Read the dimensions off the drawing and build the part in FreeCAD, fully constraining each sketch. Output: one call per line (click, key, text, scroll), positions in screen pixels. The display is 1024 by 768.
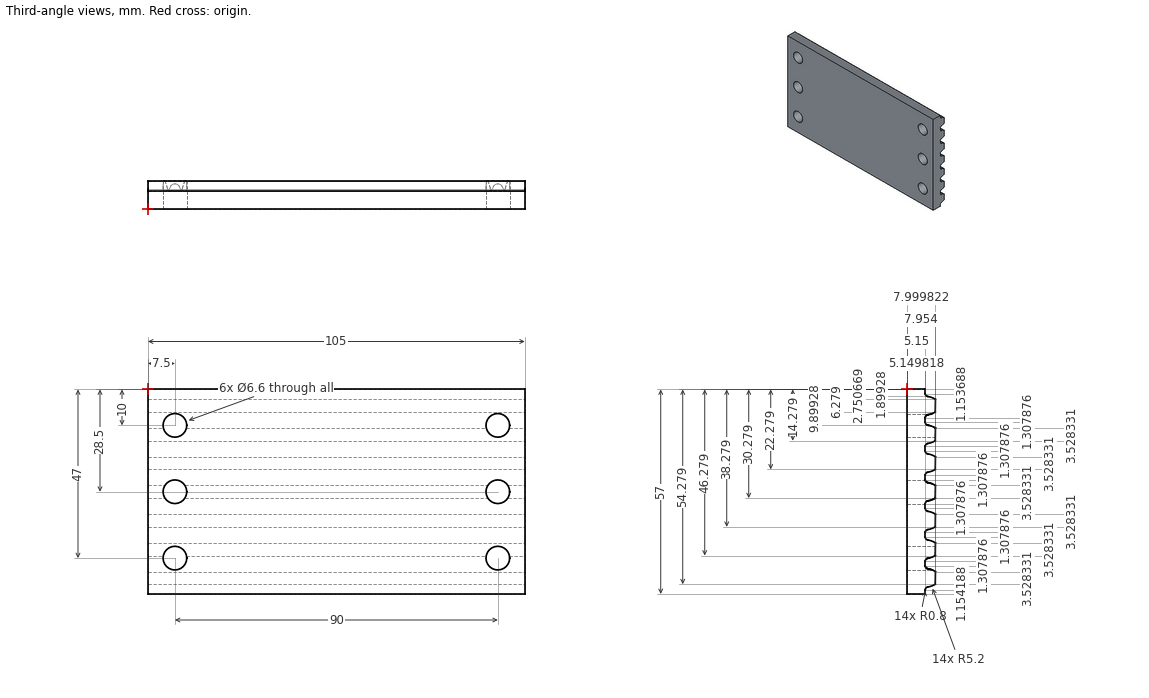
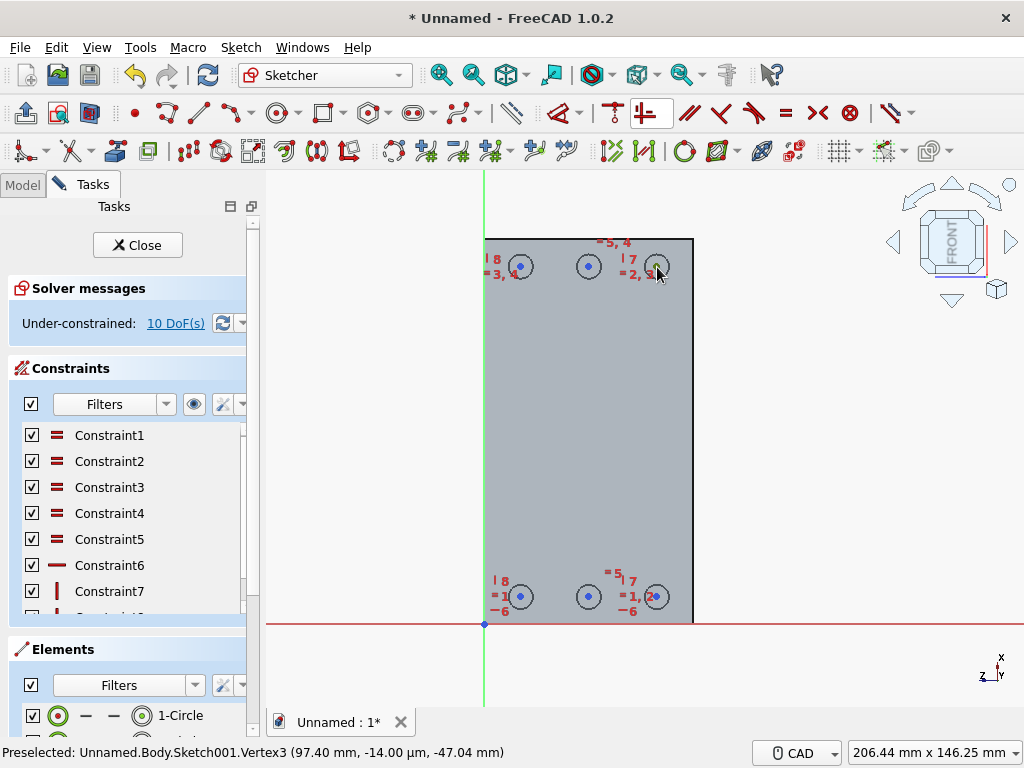
click(521, 267)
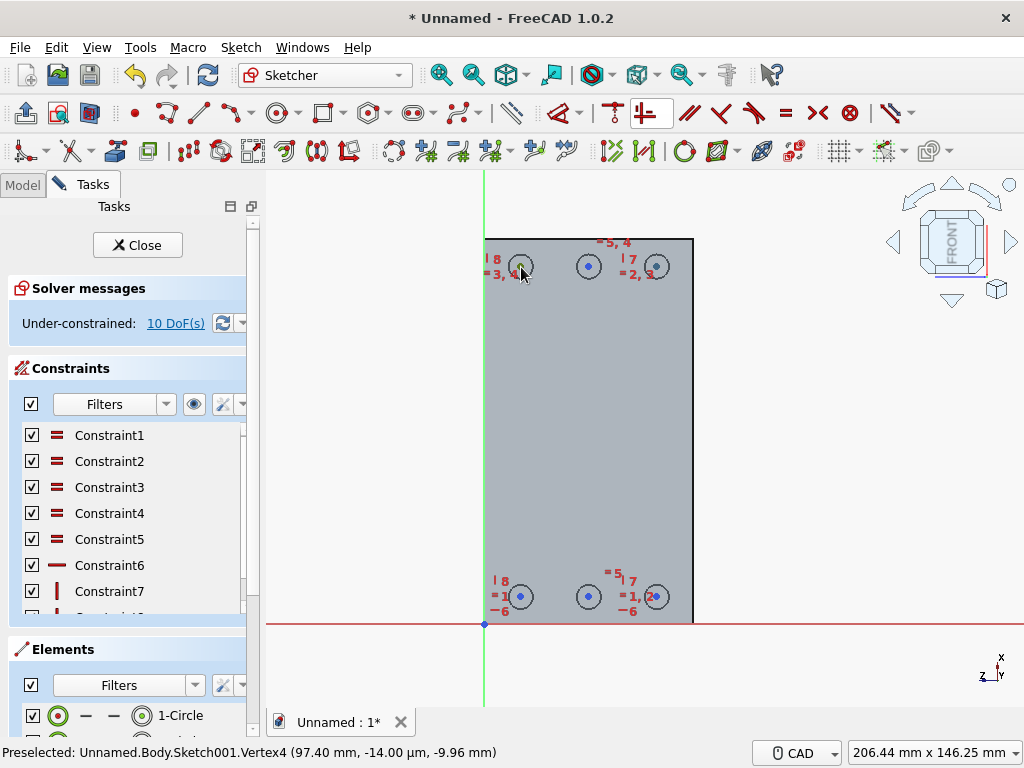
click(668, 114)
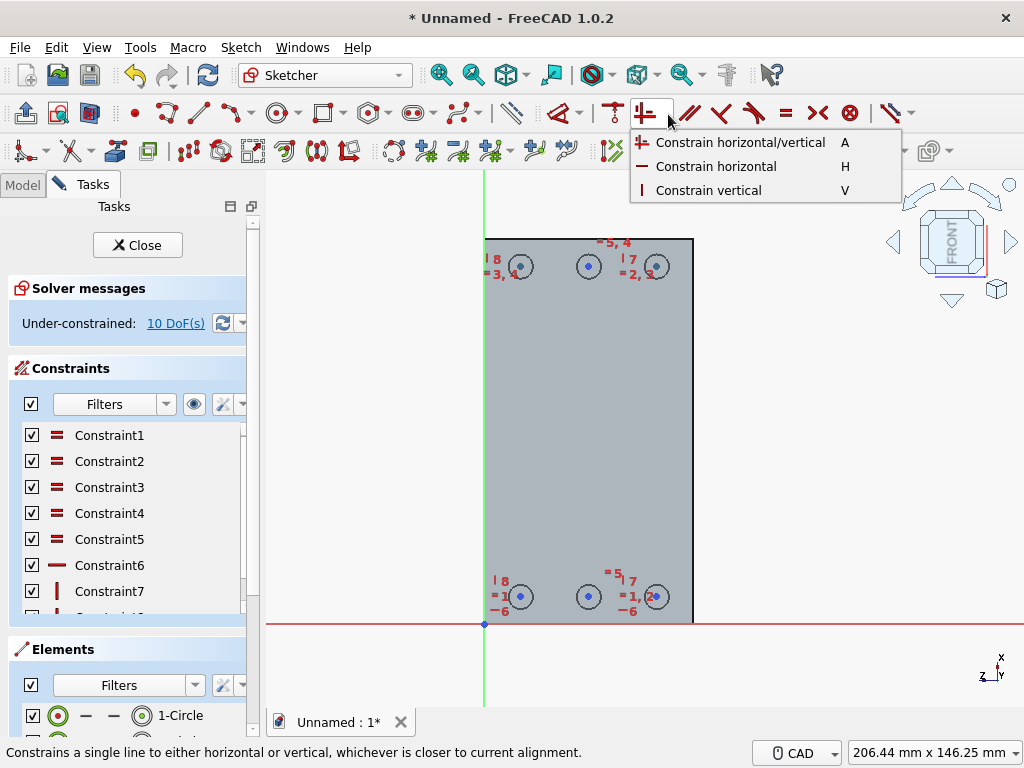
click(766, 166)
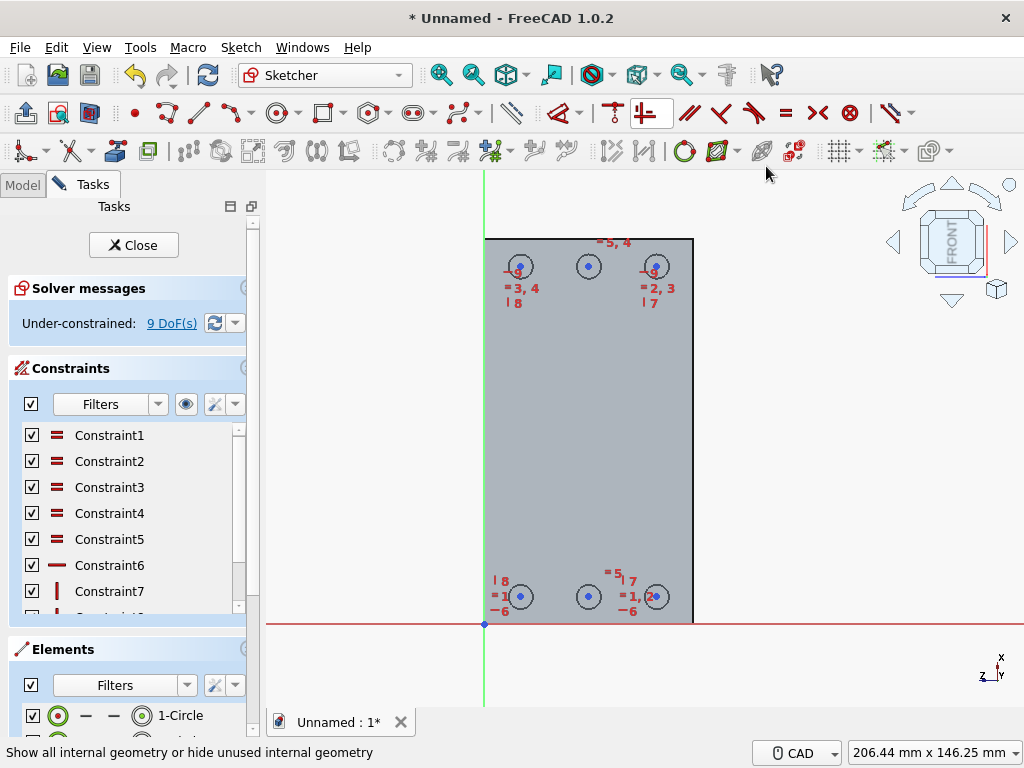
click(657, 267)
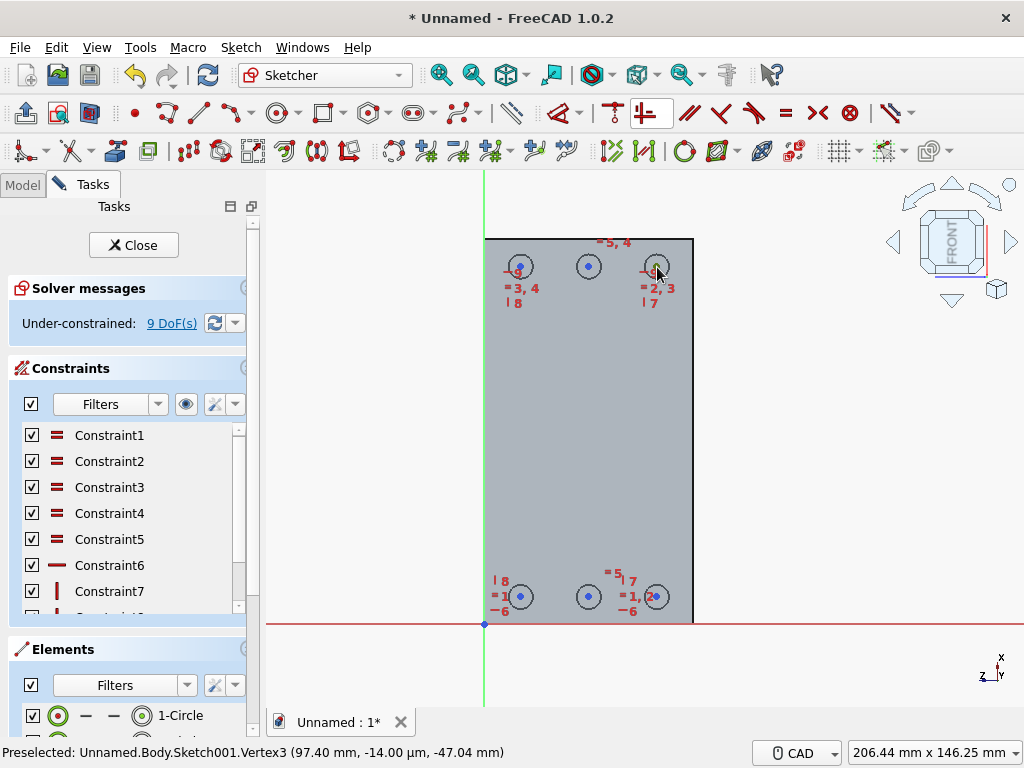
click(589, 267)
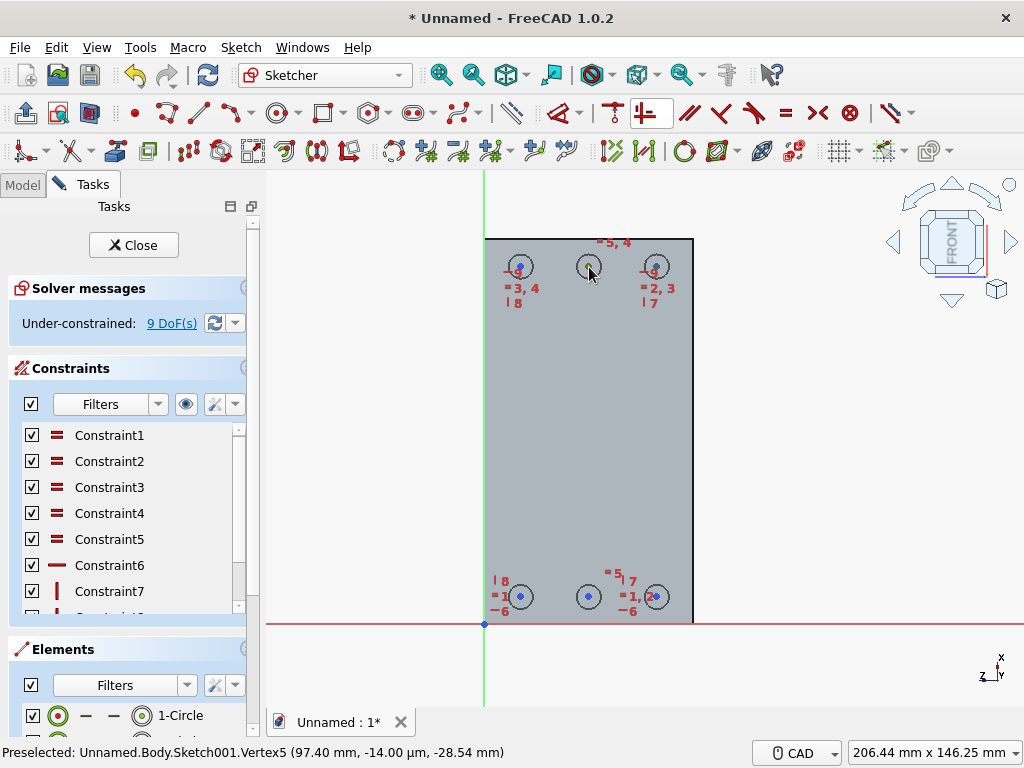
key(h)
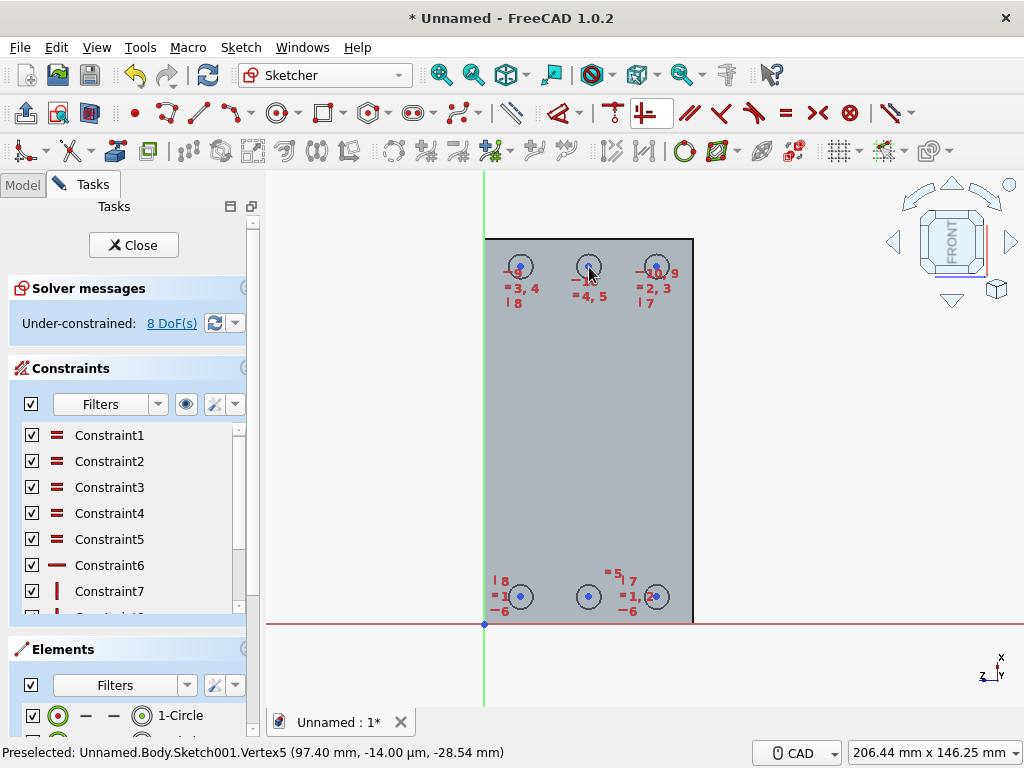
click(589, 267)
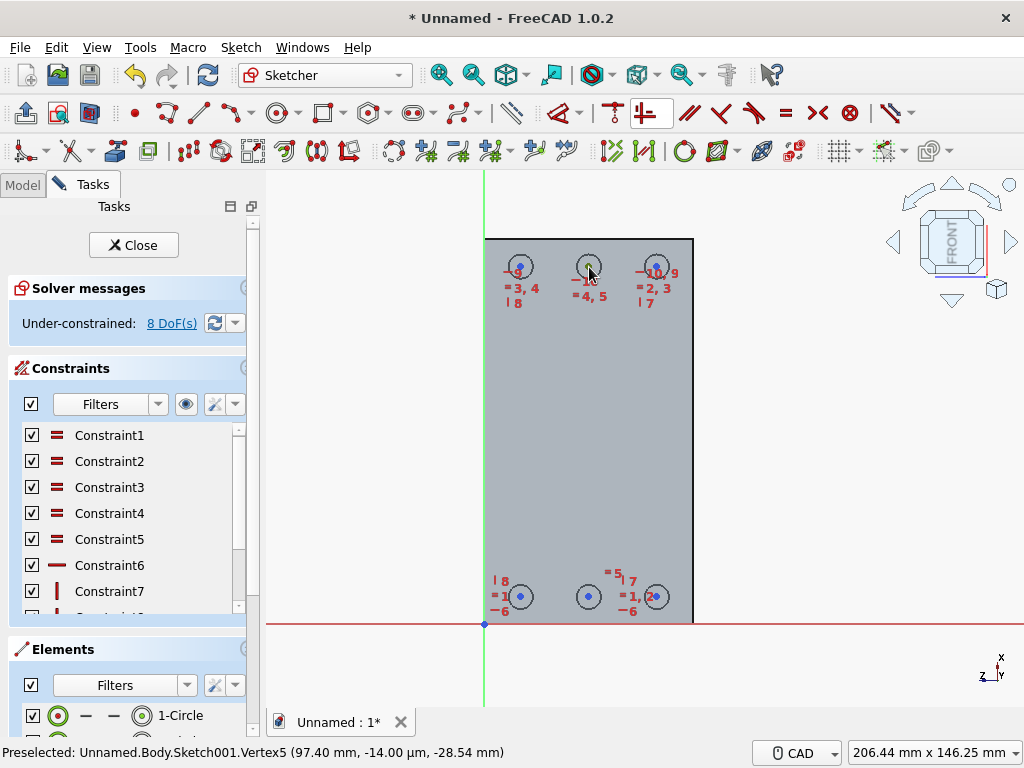
click(589, 597)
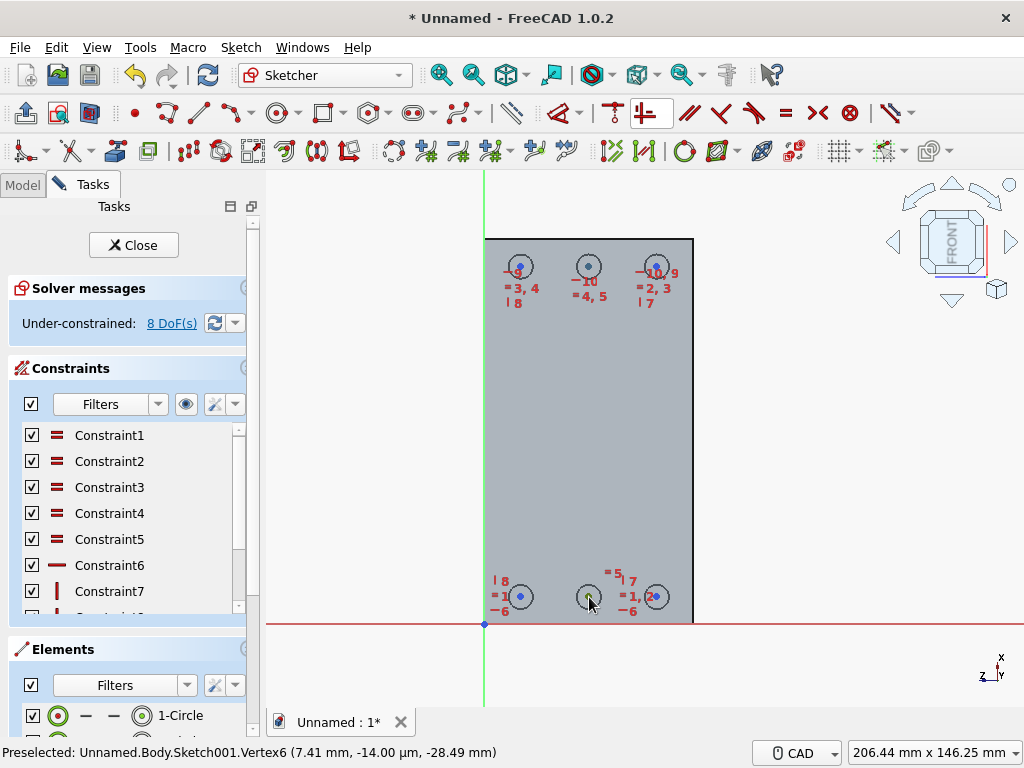
click(668, 114)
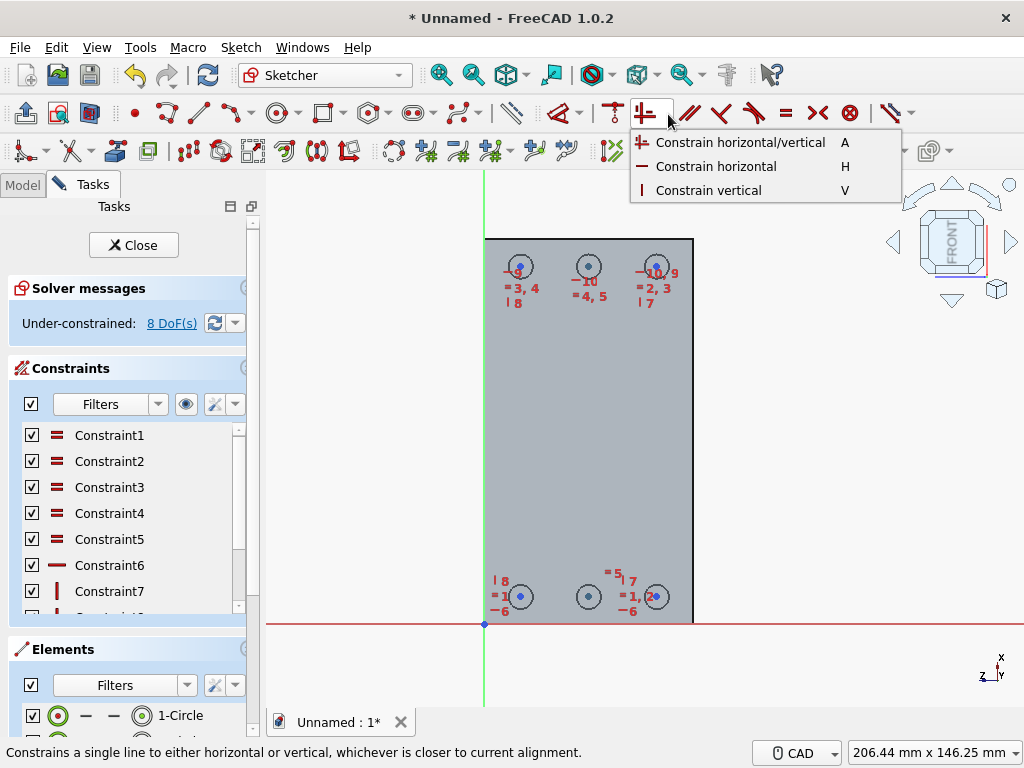
click(766, 190)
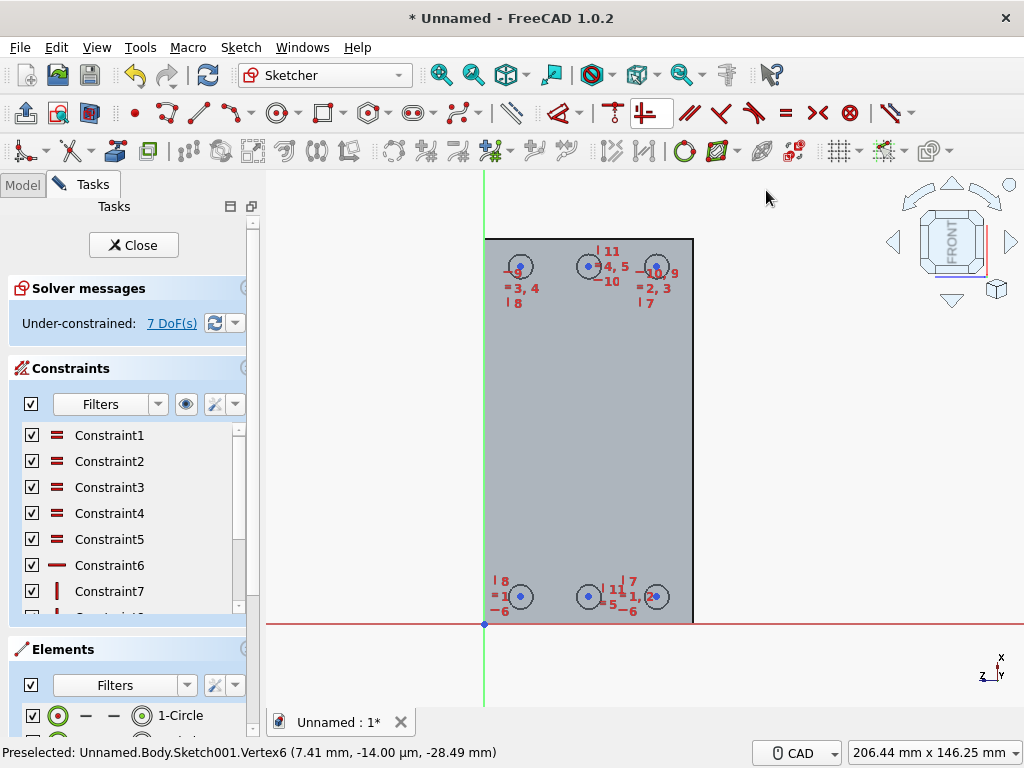
click(521, 597)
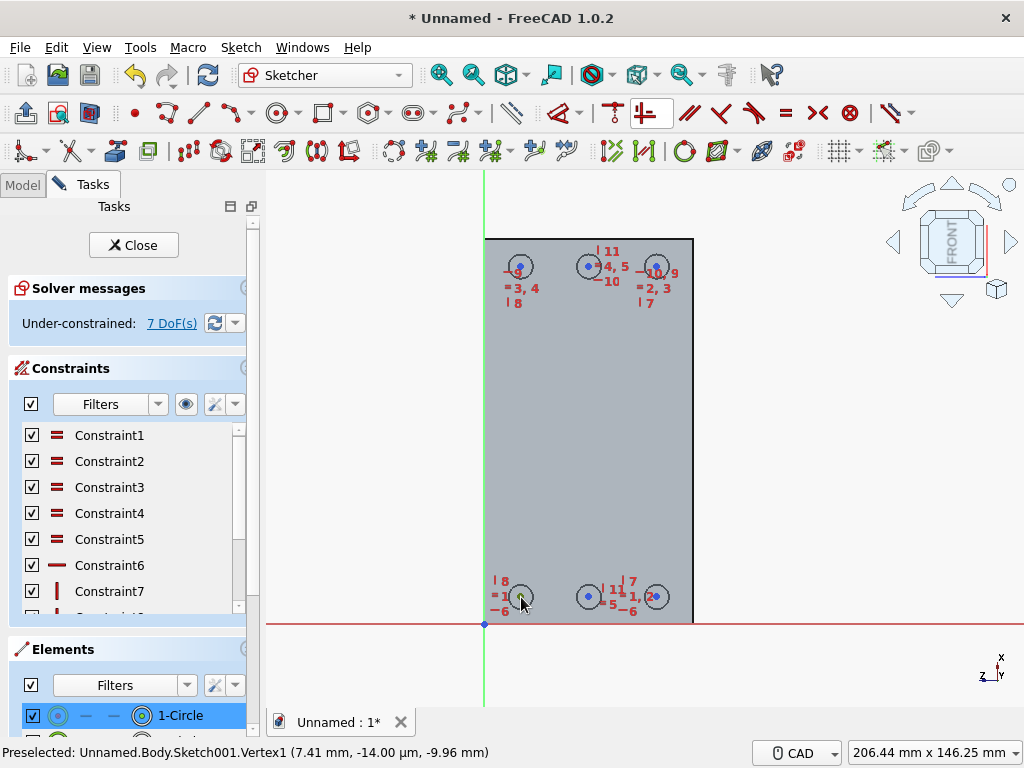
click(589, 597)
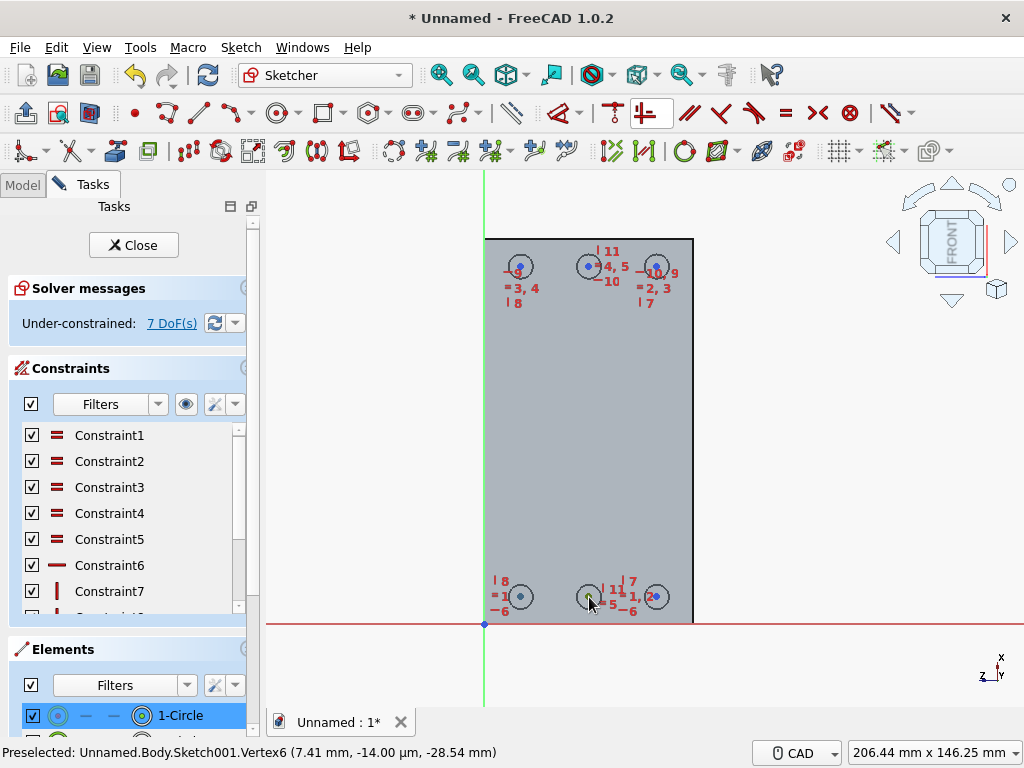
click(668, 114)